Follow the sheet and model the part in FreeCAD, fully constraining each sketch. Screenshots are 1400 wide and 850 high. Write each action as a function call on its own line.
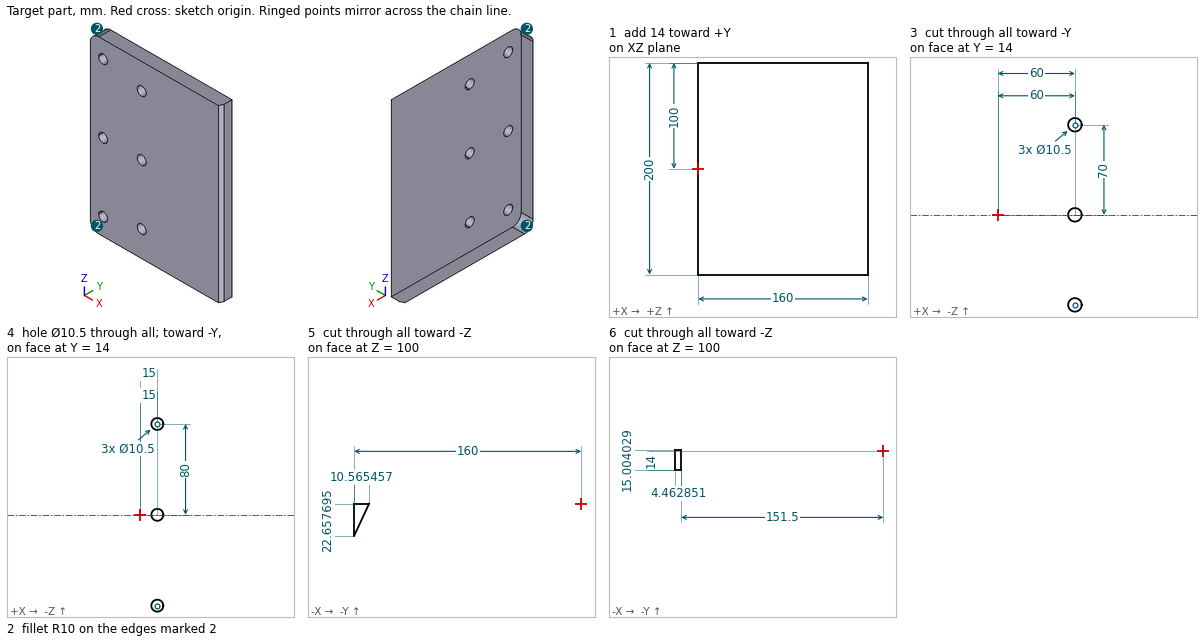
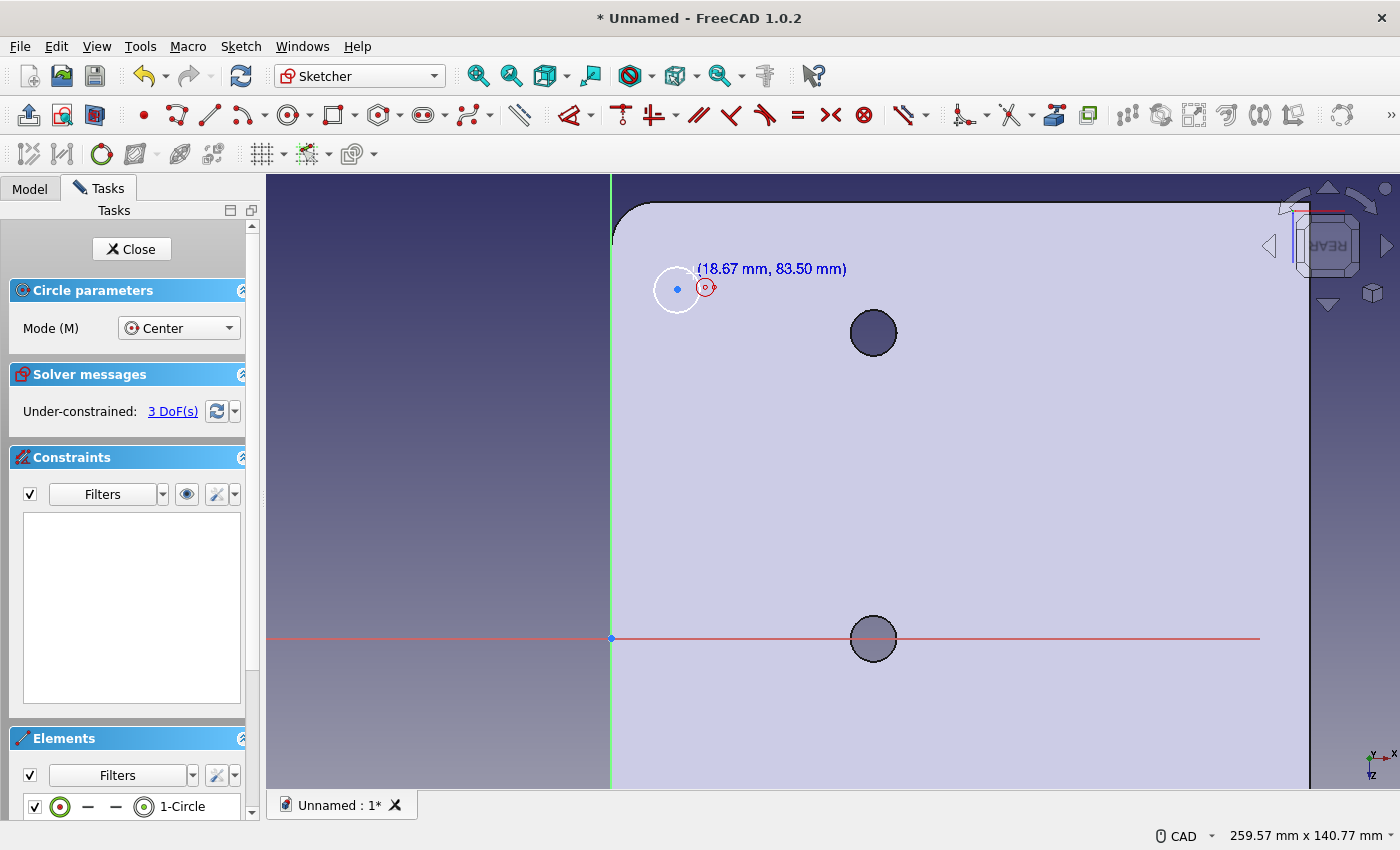
scroll(897, 290, down, 3)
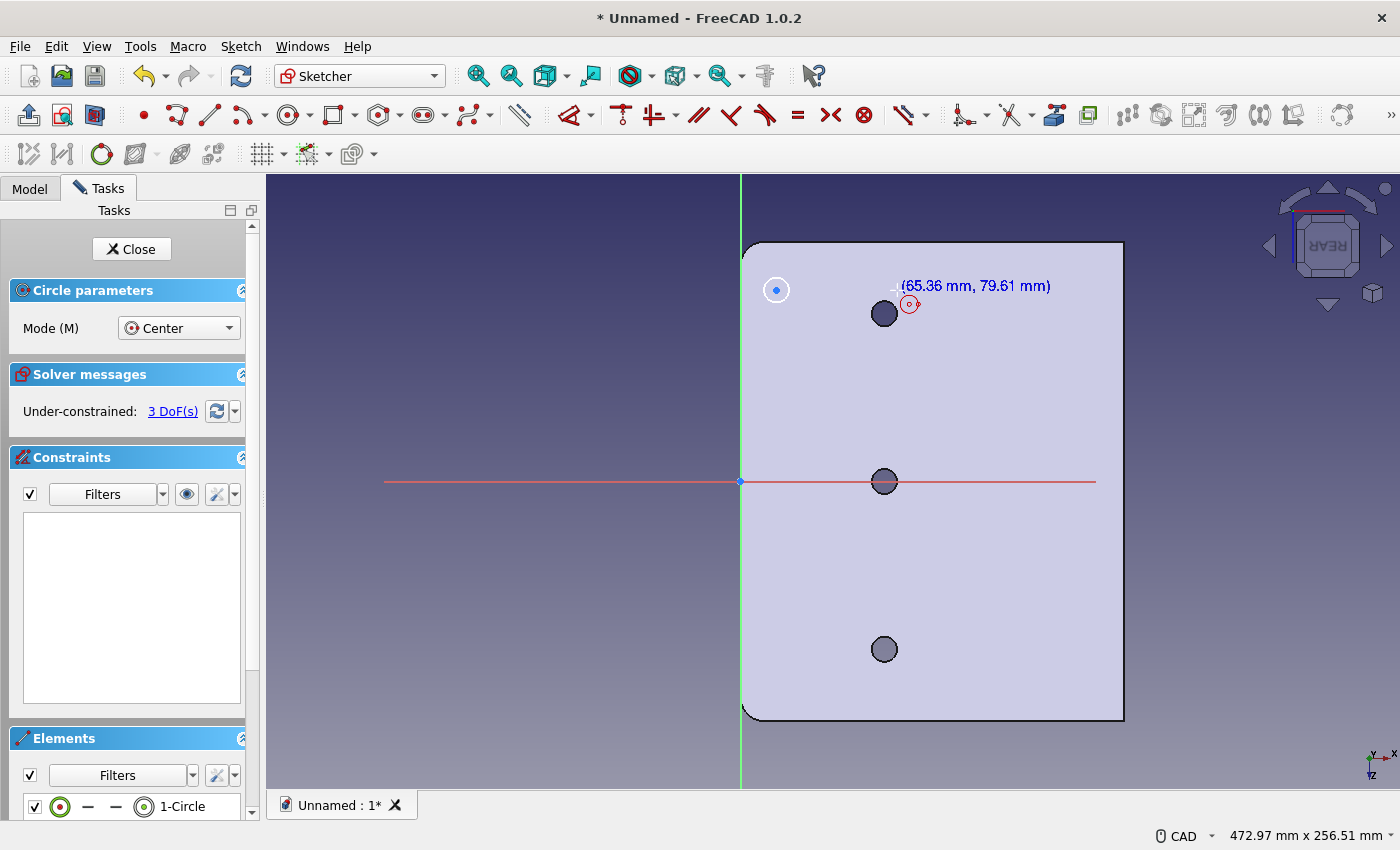
scroll(777, 673, up, 3)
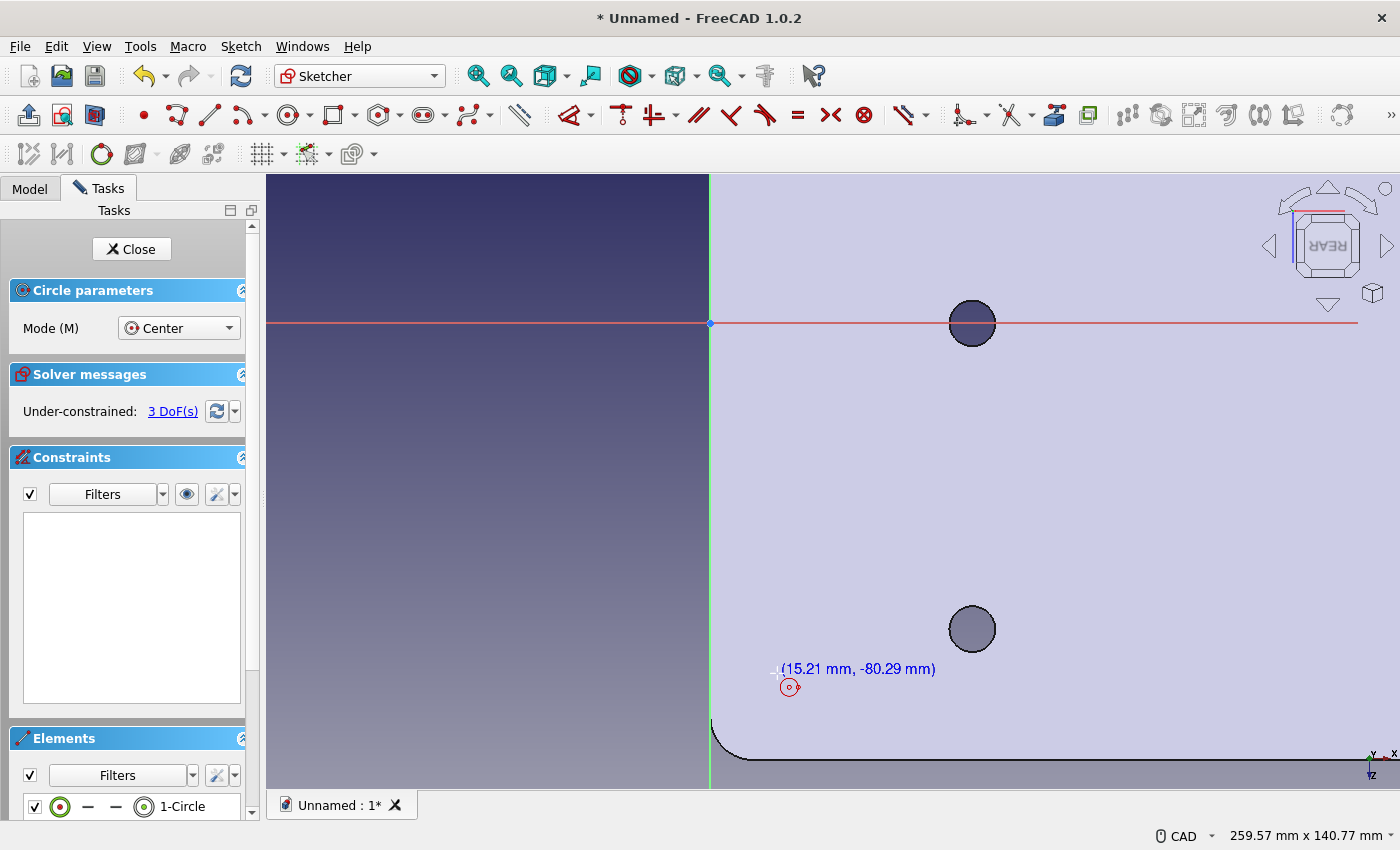
click(776, 673)
click(792, 657)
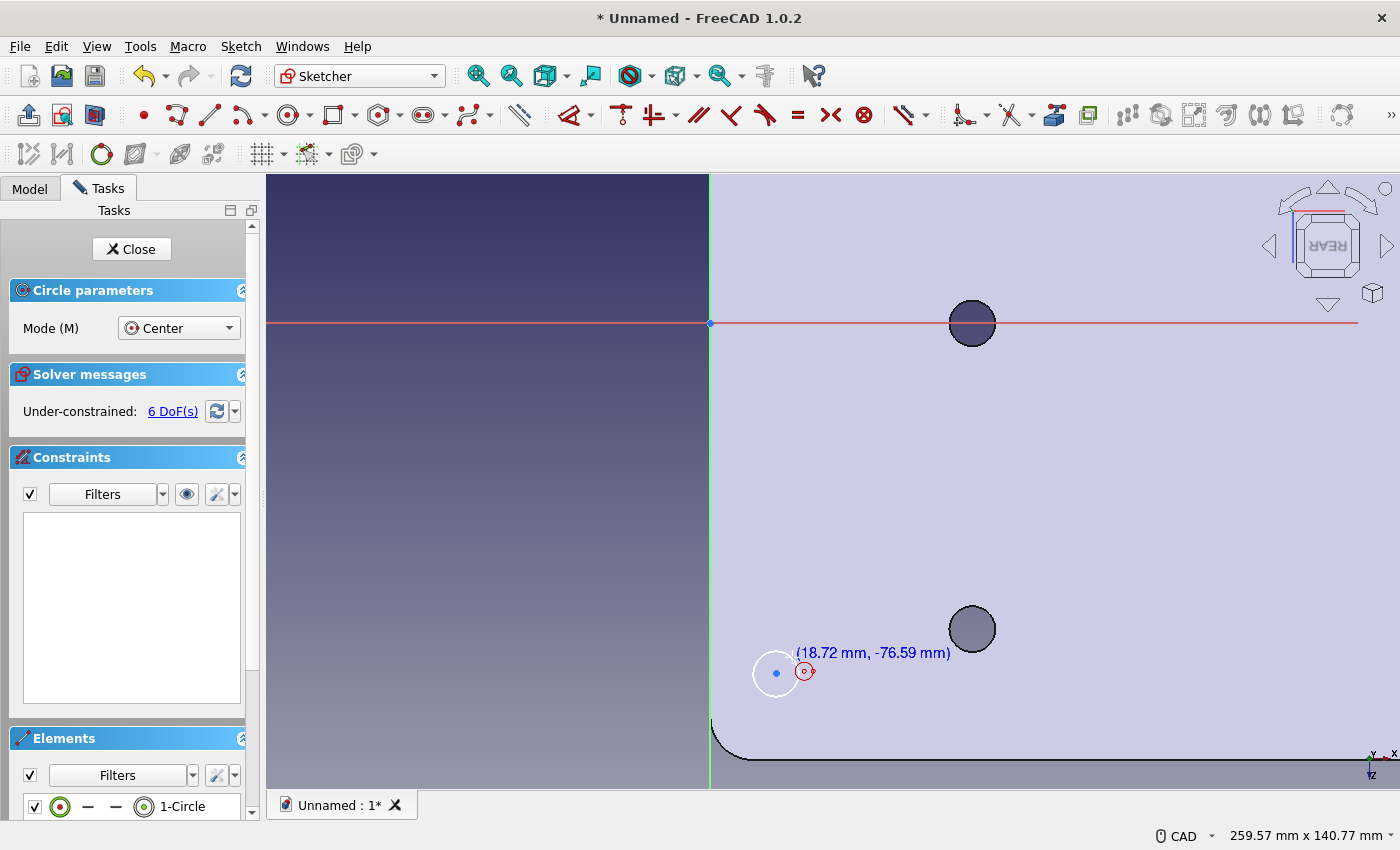
click(776, 323)
click(792, 307)
key(Escape)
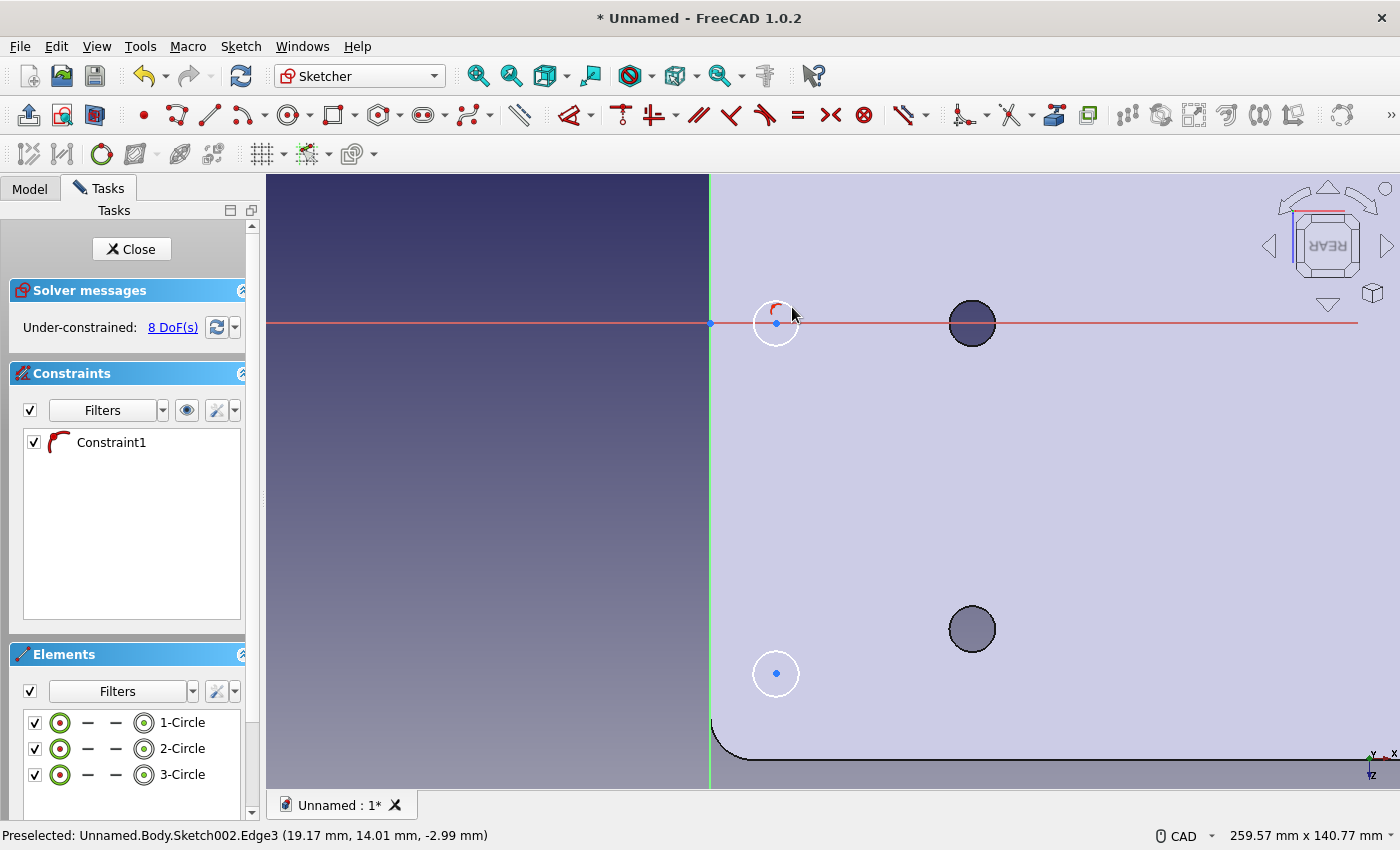
scroll(777, 674, down, 3)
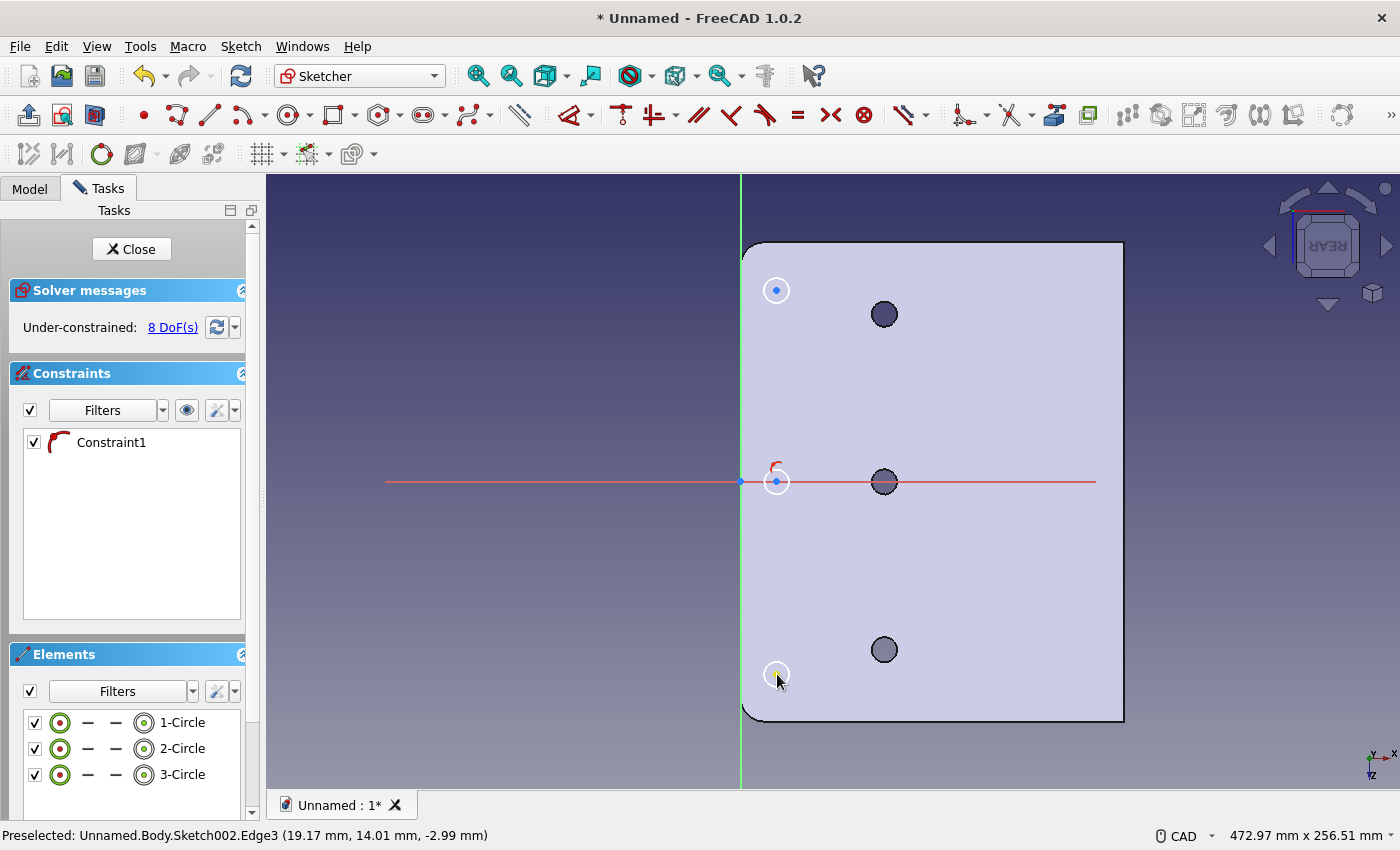
click(785, 282)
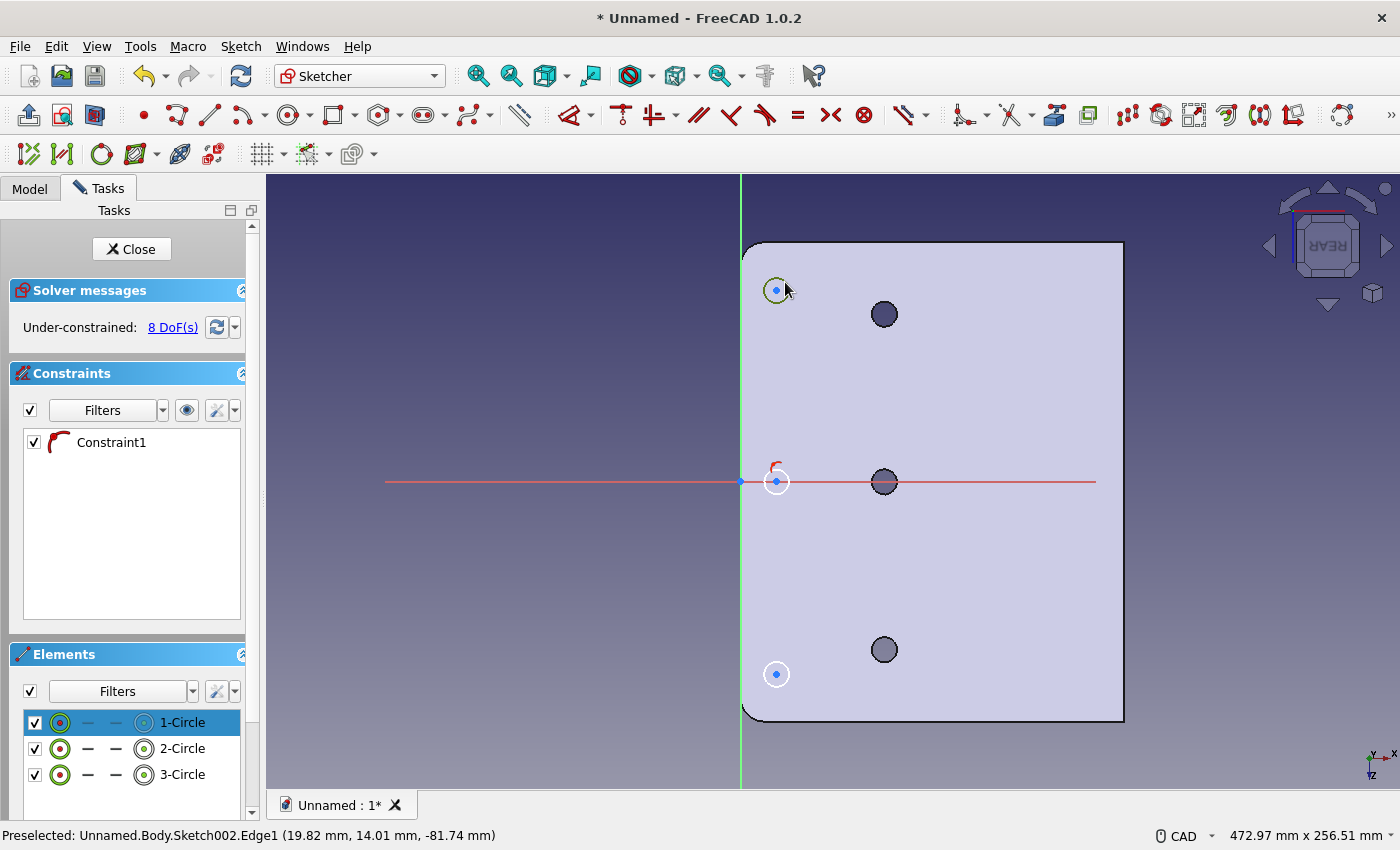
click(785, 666)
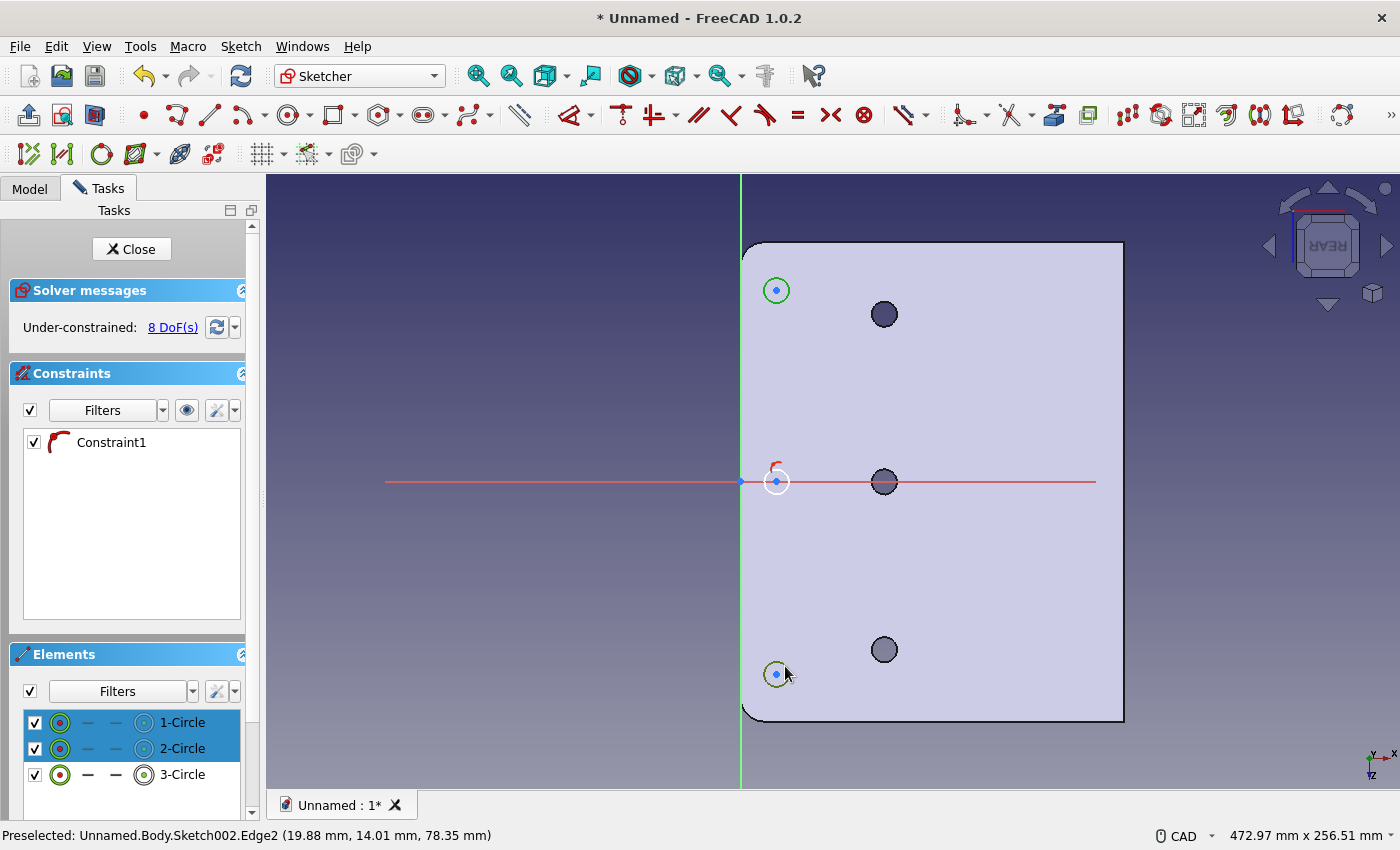
click(764, 482)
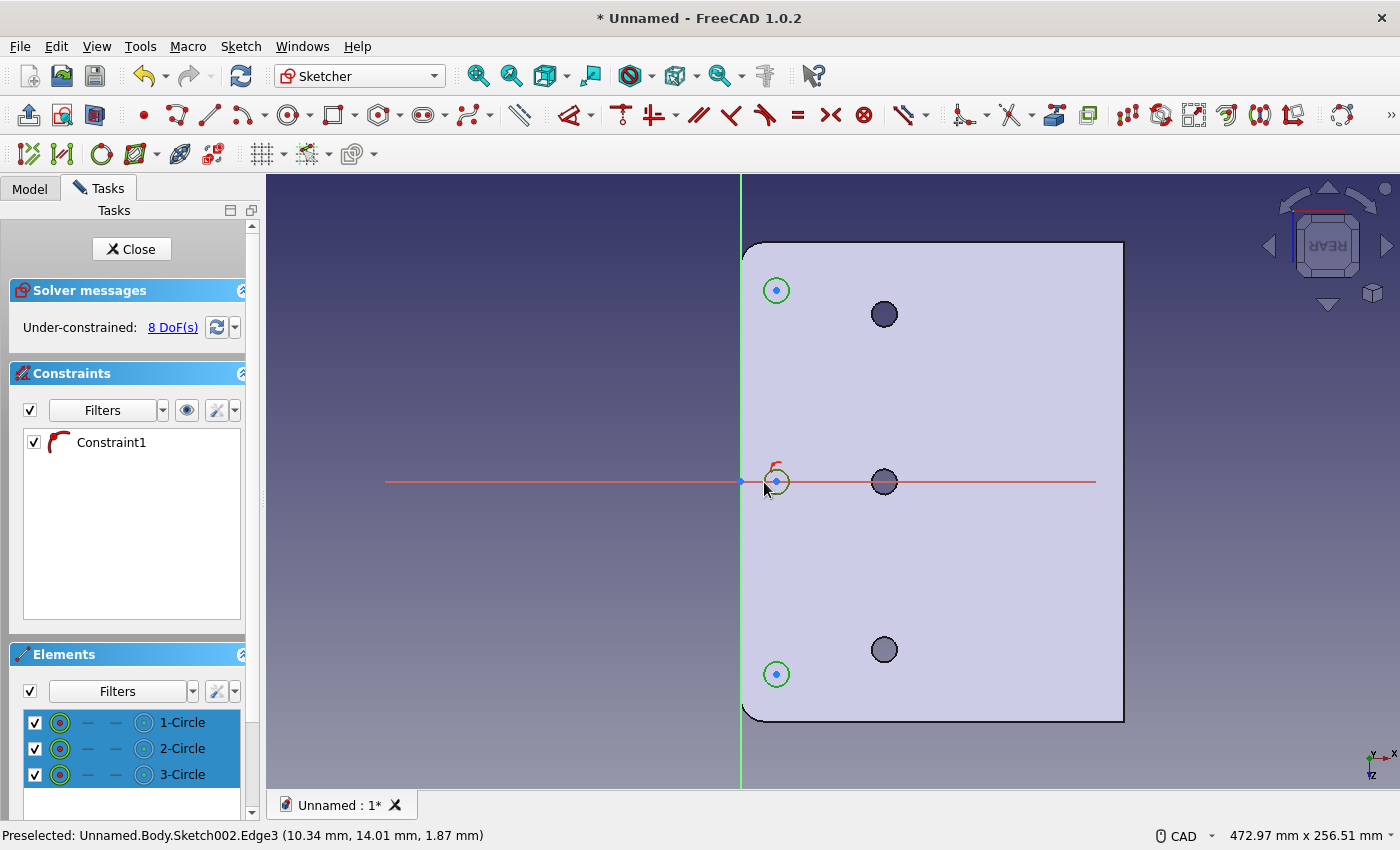
key(e)